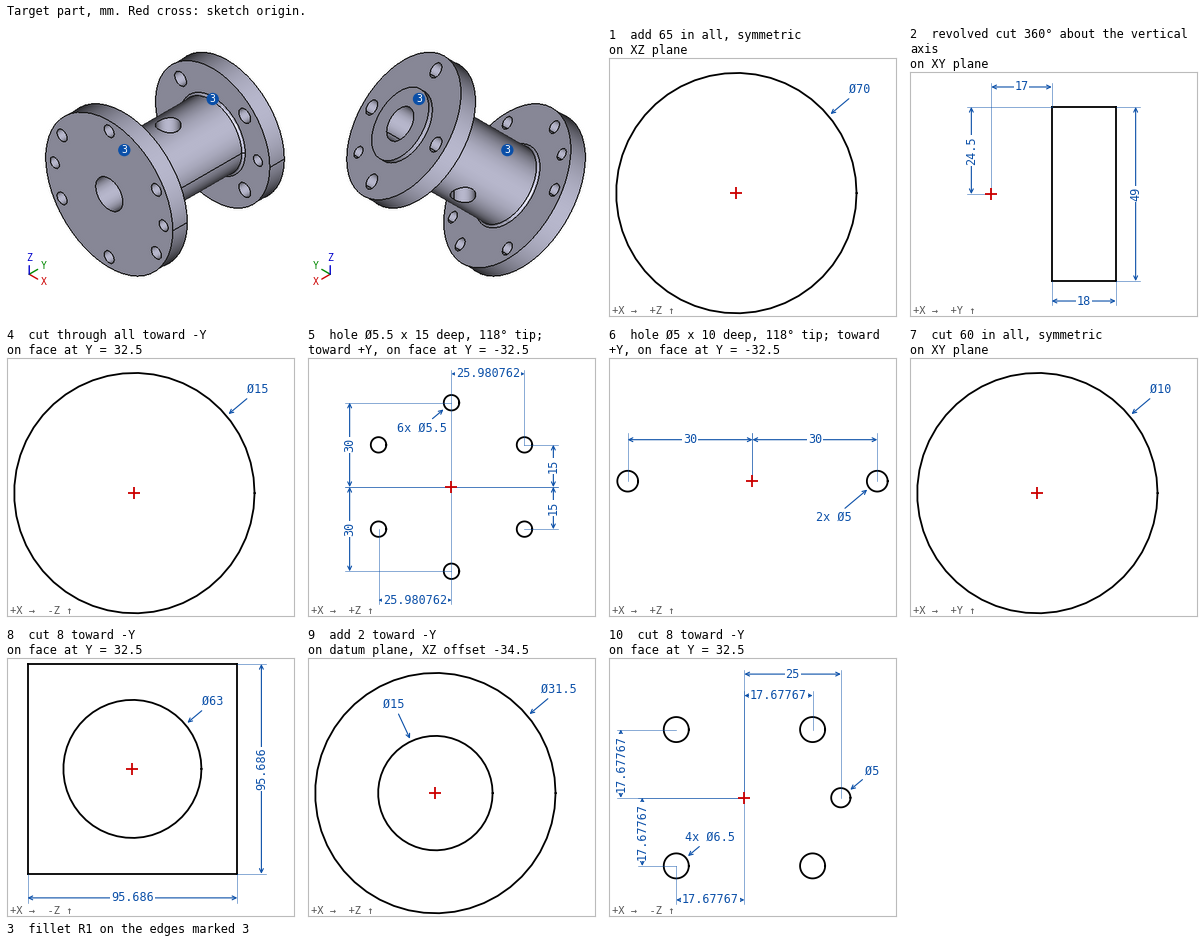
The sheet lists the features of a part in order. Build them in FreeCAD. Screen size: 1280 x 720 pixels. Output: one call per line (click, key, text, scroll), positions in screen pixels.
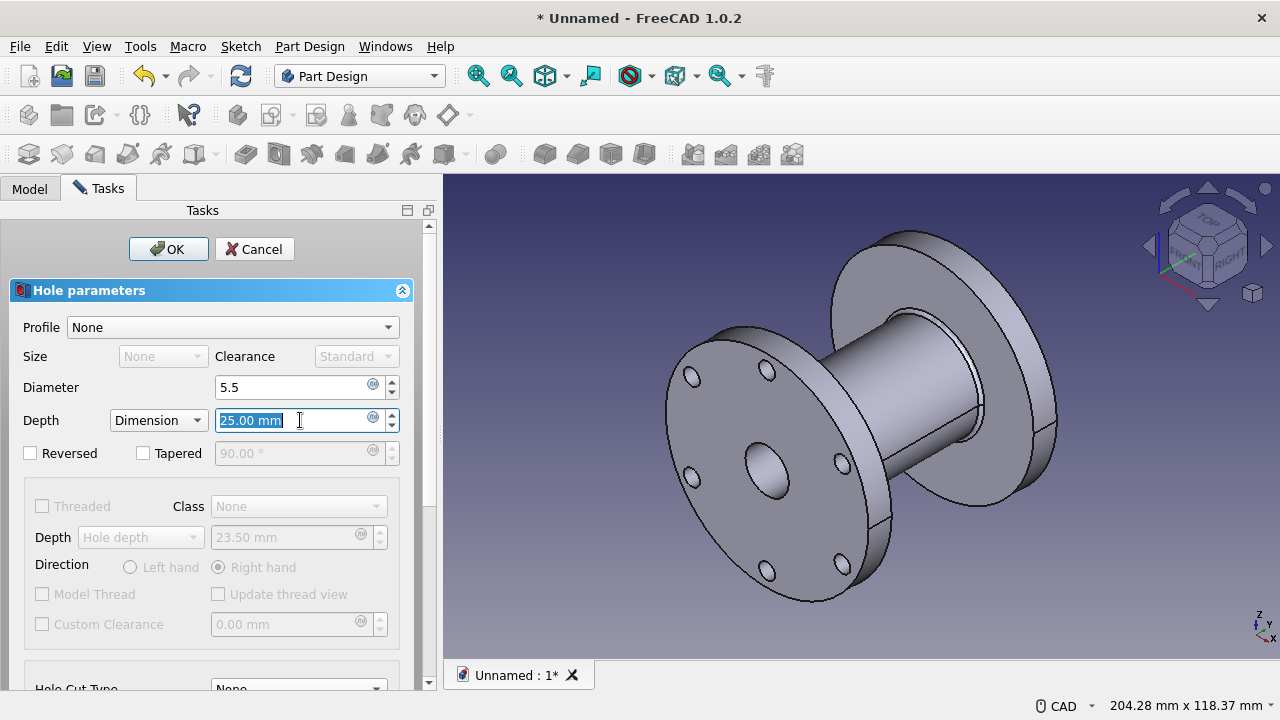
text(15)
key(Tab)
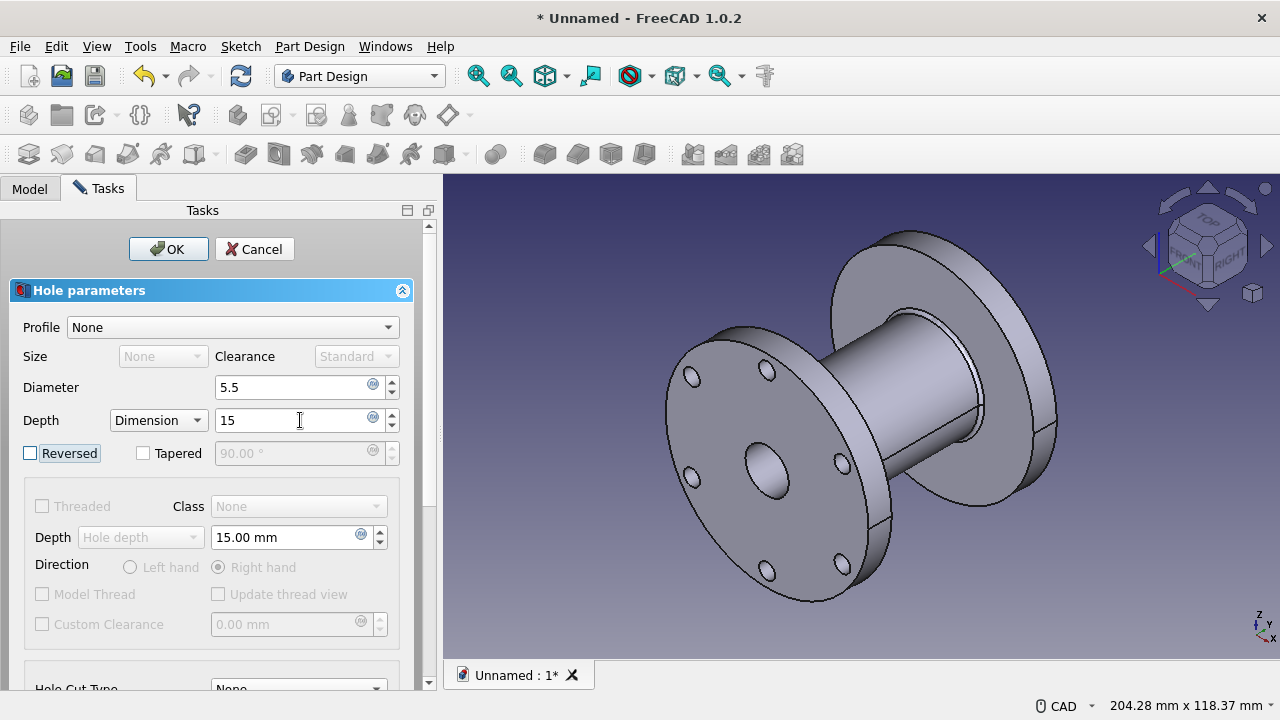
click(169, 249)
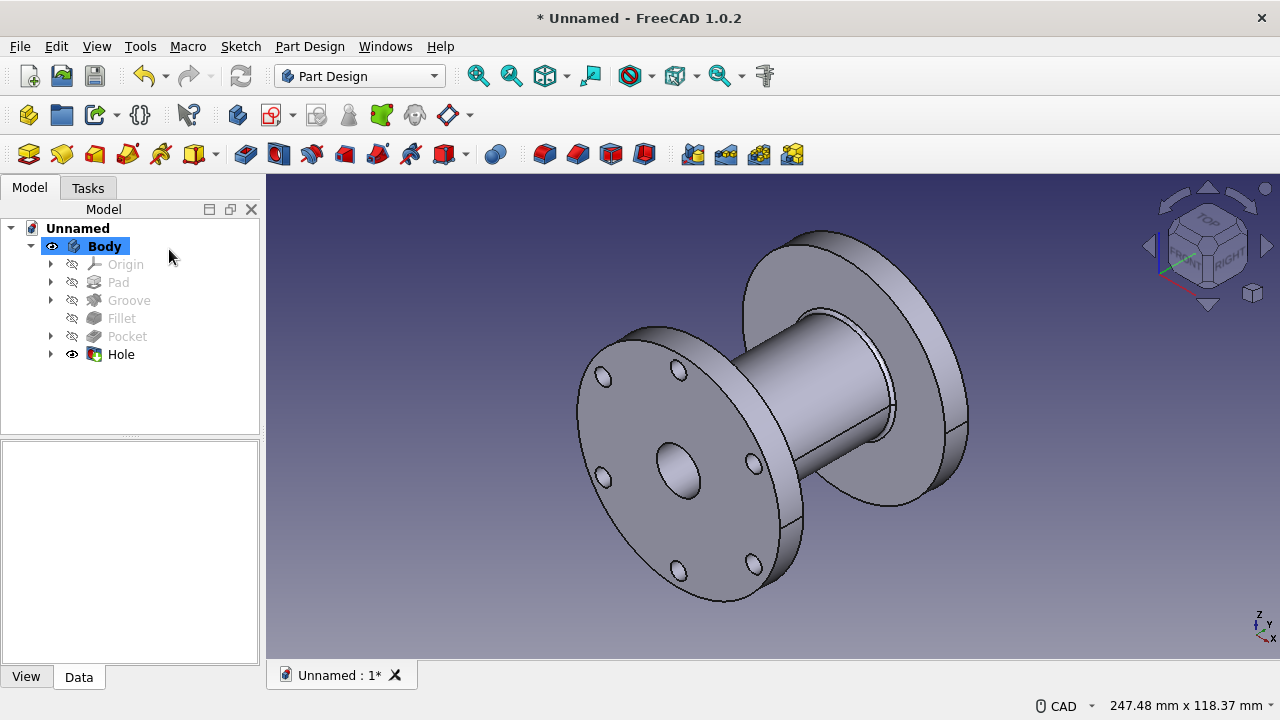
click(737, 503)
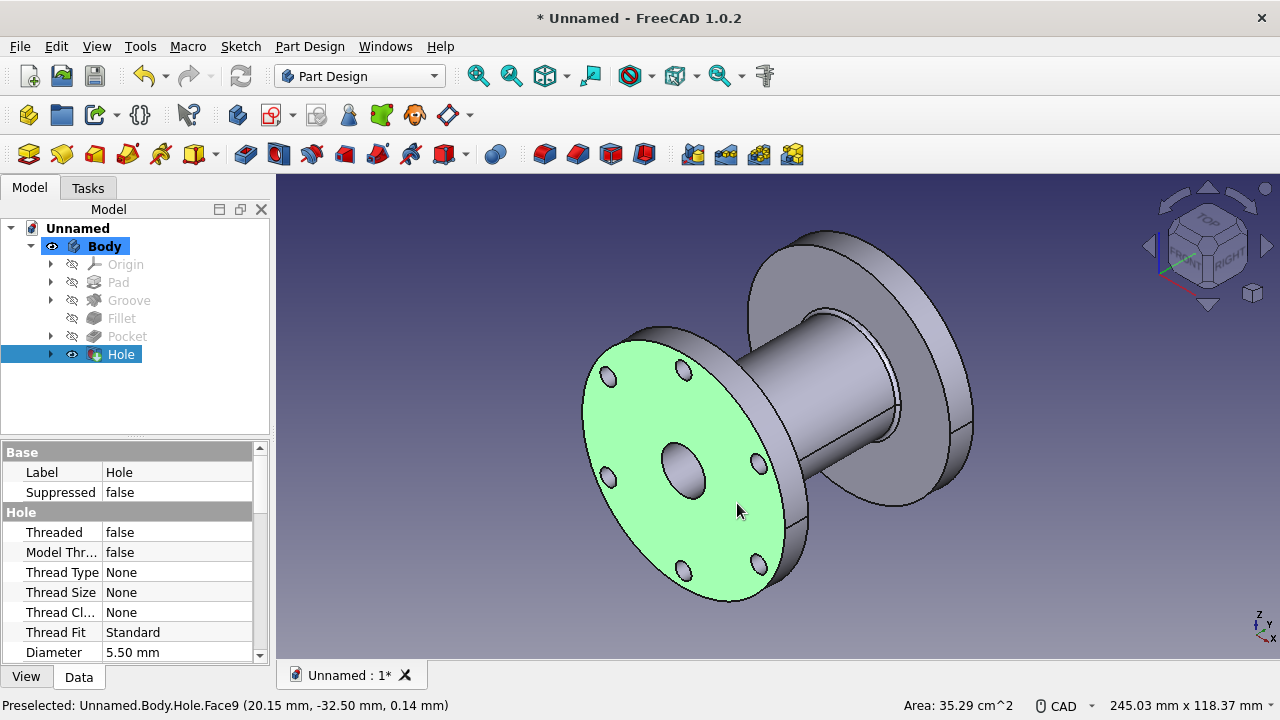
click(270, 116)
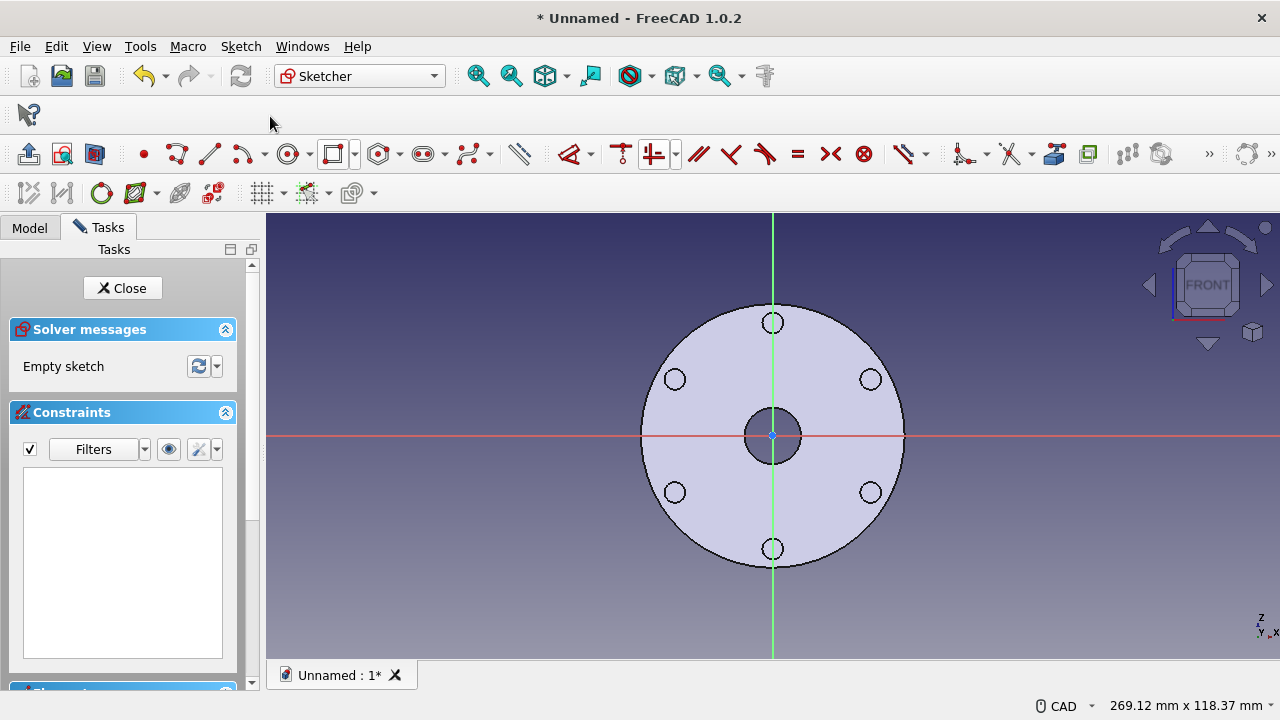
scroll(829, 436, up, 4)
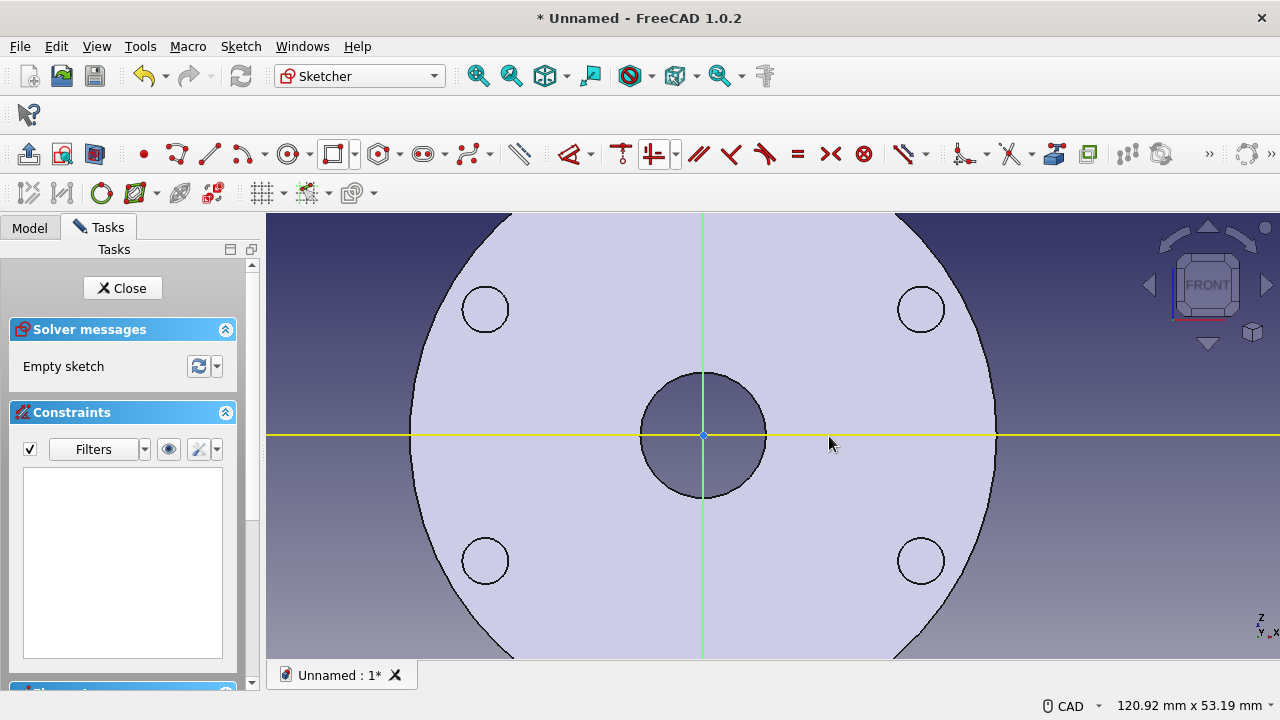
click(288, 154)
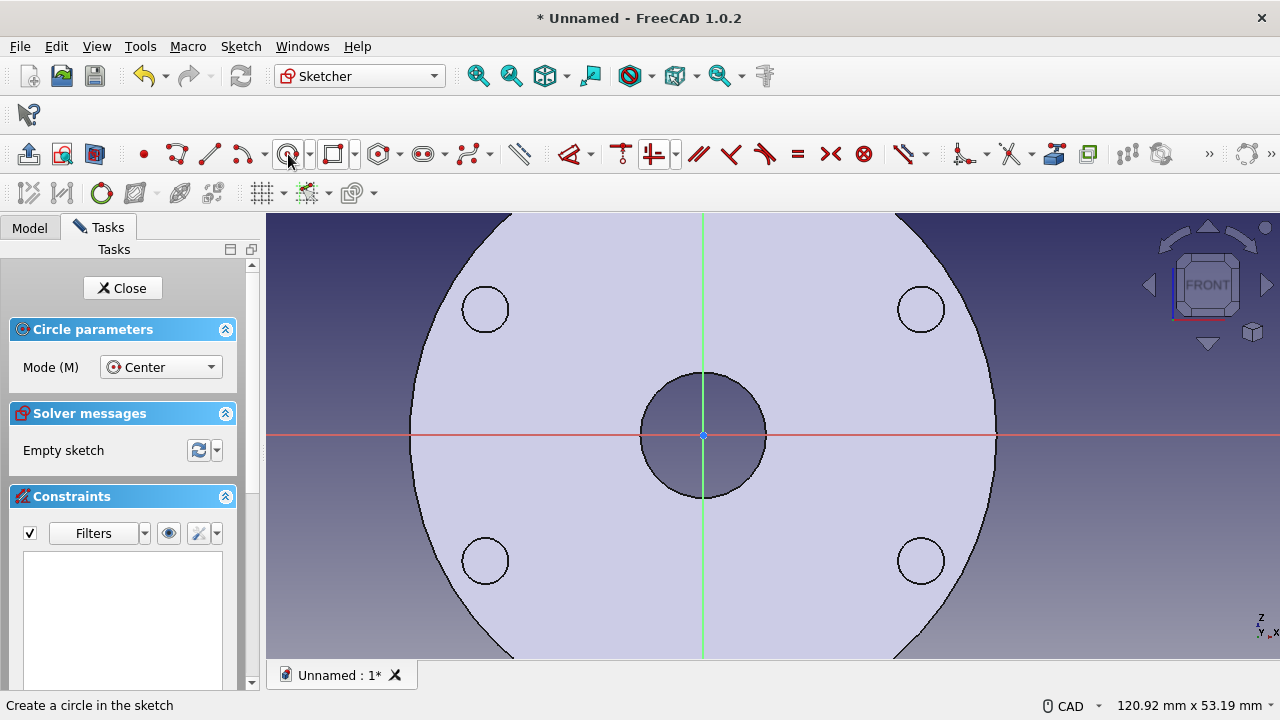
click(955, 435)
move(970, 420)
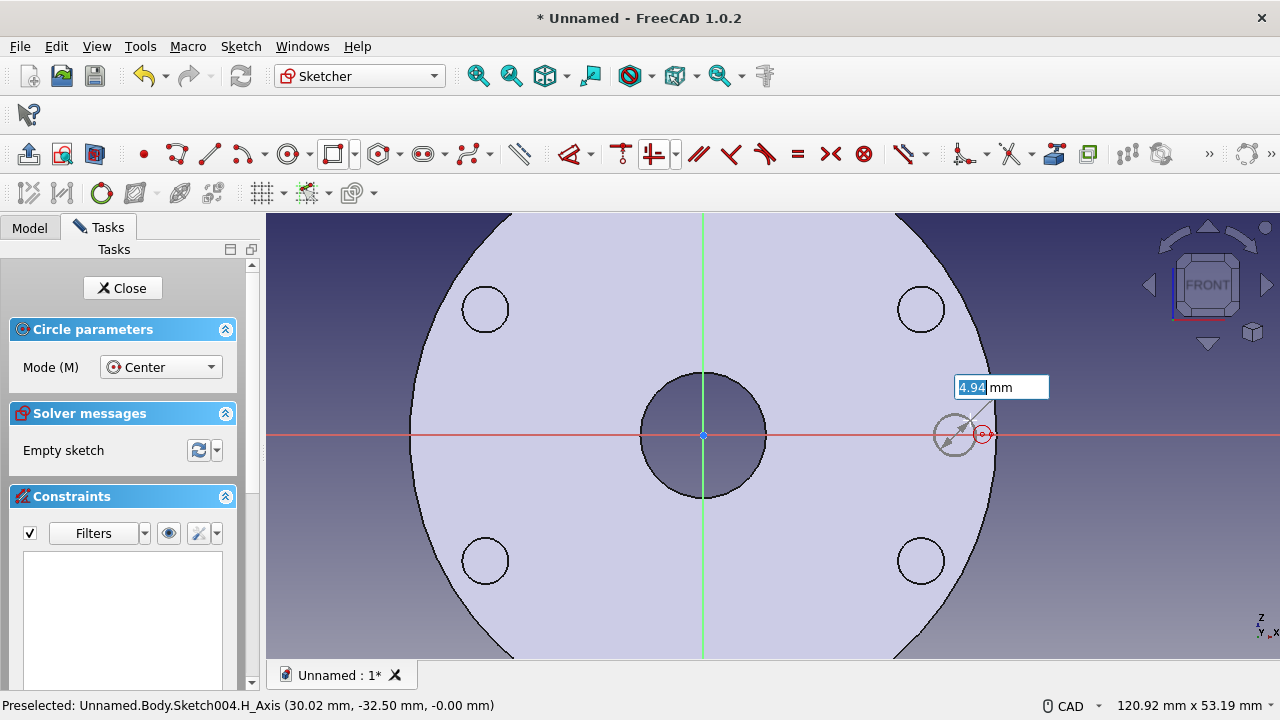
text(5)
key(Return)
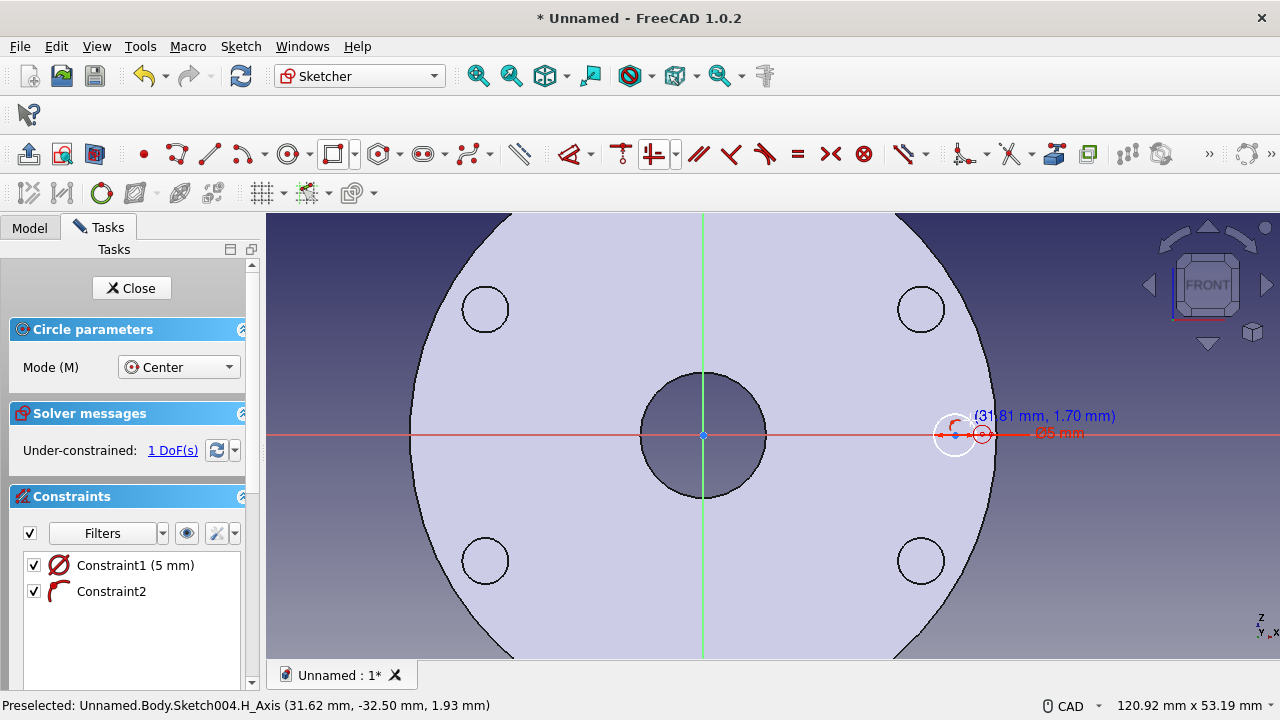
click(452, 435)
move(466, 420)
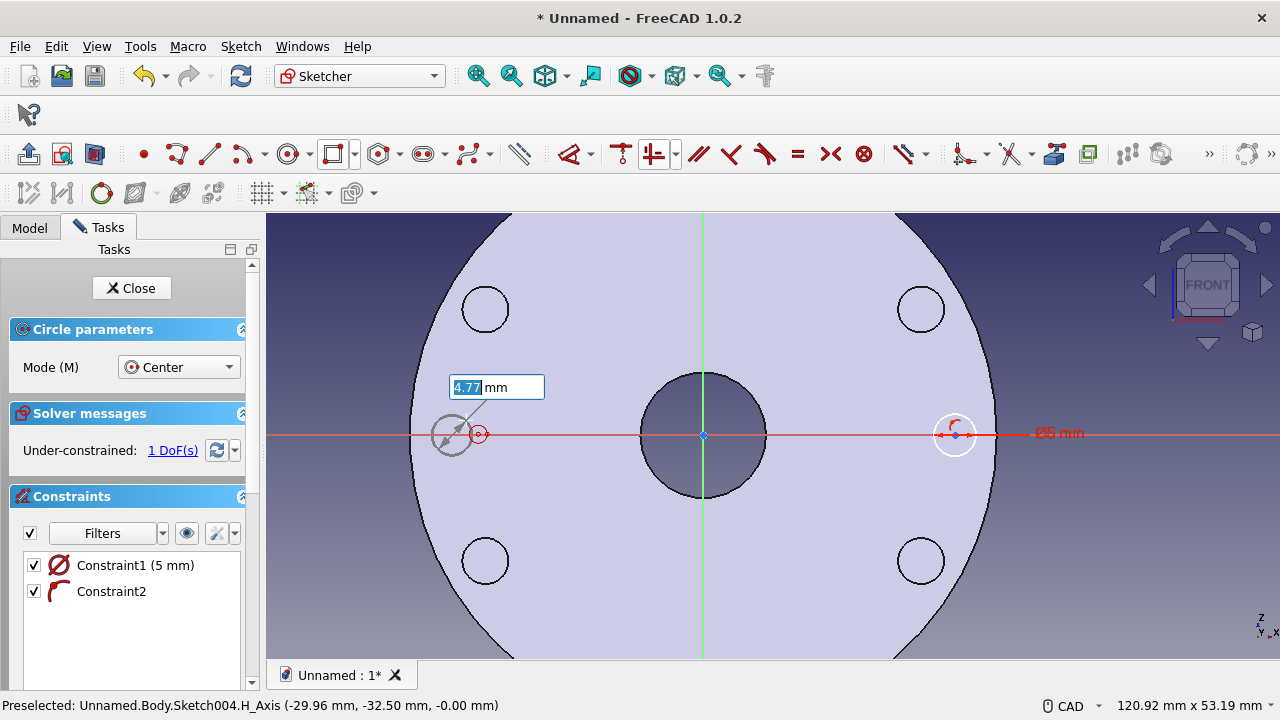
text(5)
key(Return)
key(Escape)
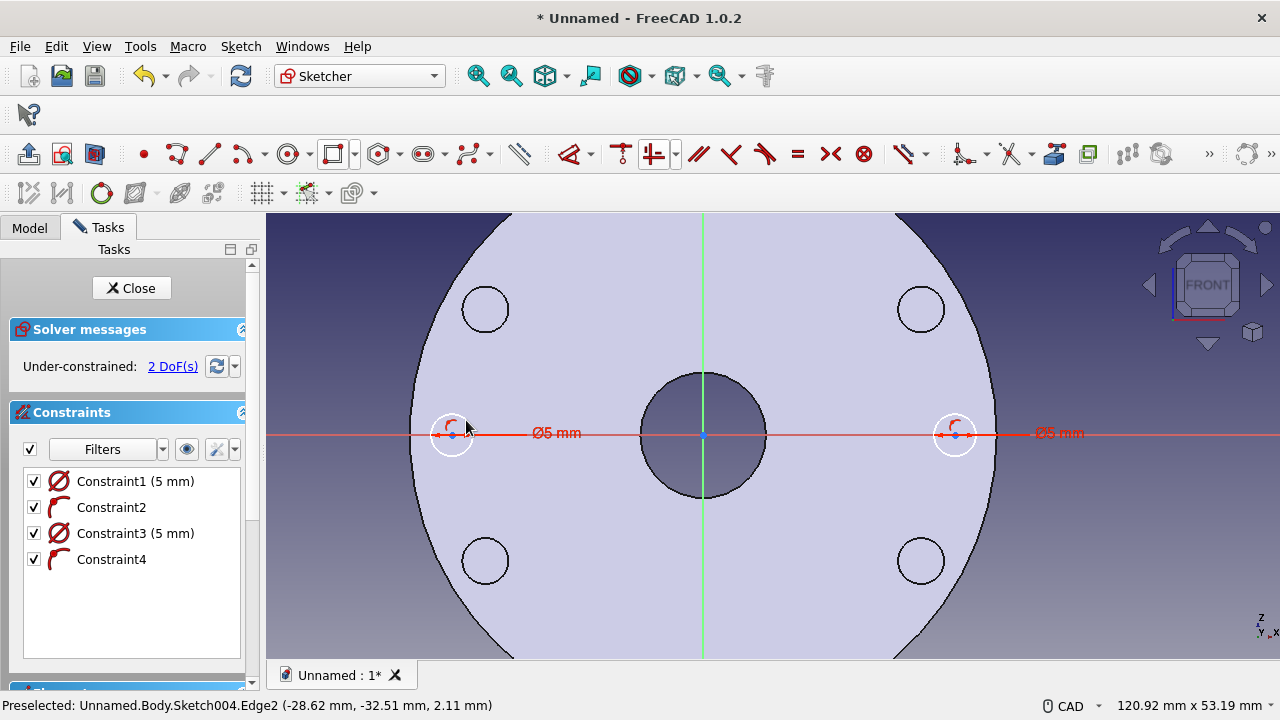
click(568, 154)